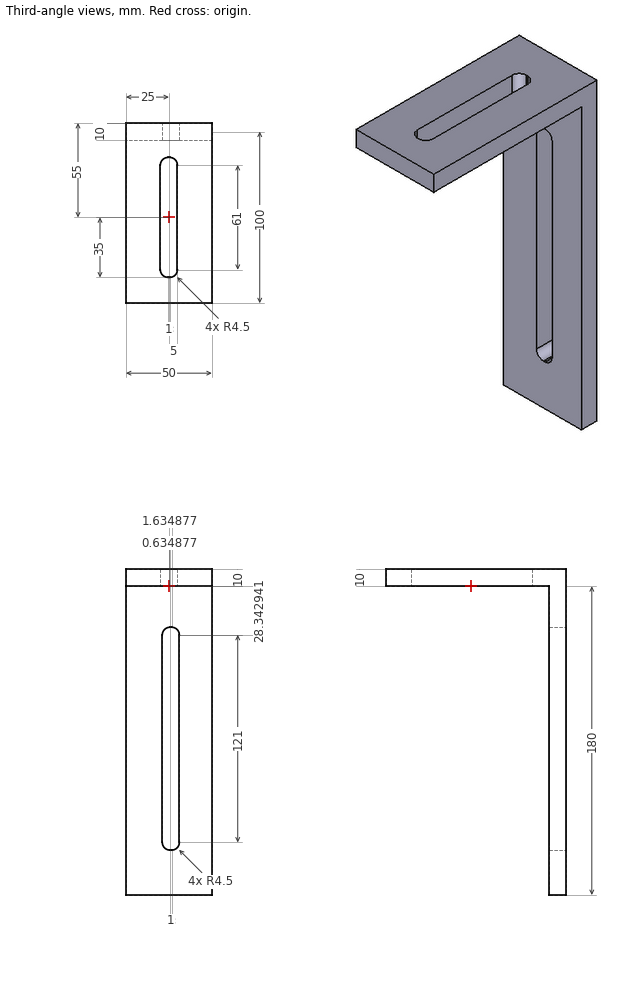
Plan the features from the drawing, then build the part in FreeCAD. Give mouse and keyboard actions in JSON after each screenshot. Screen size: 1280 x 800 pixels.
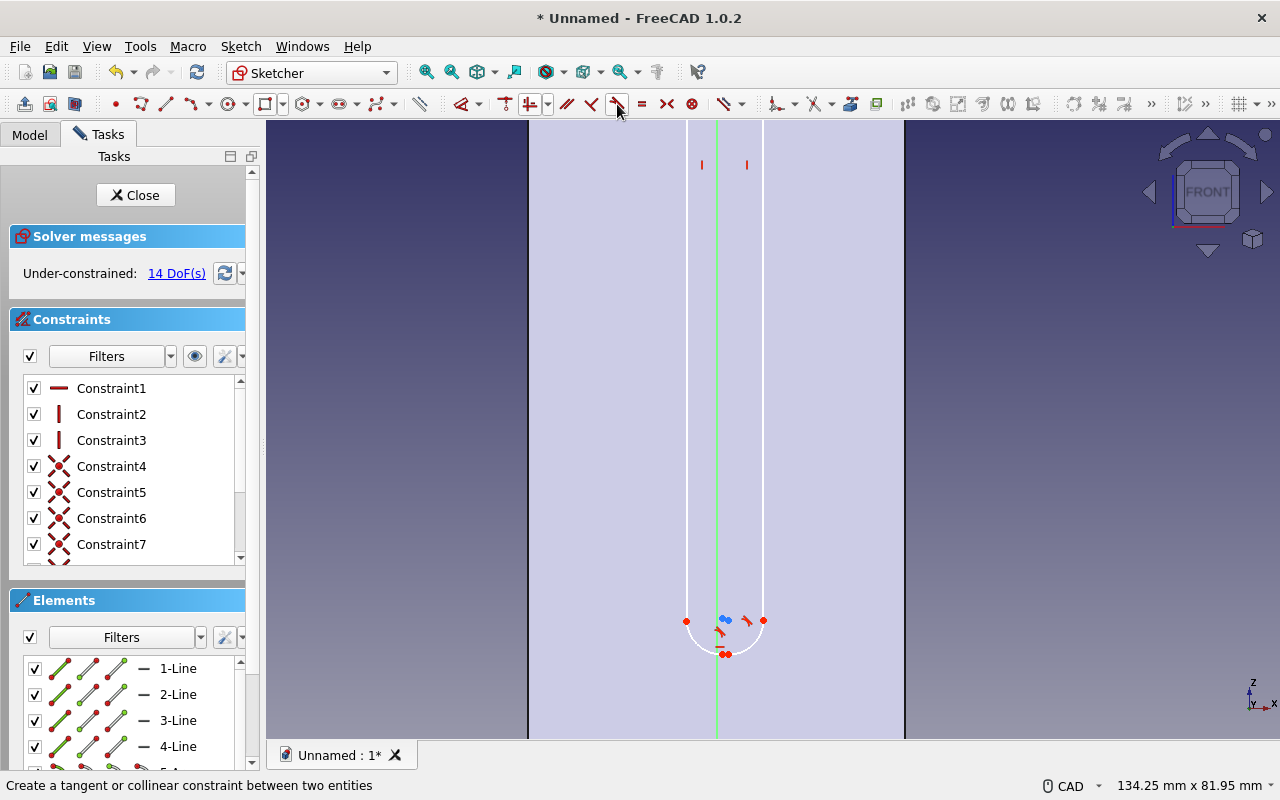
{"action": "left_click", "coordinate": [763, 347]}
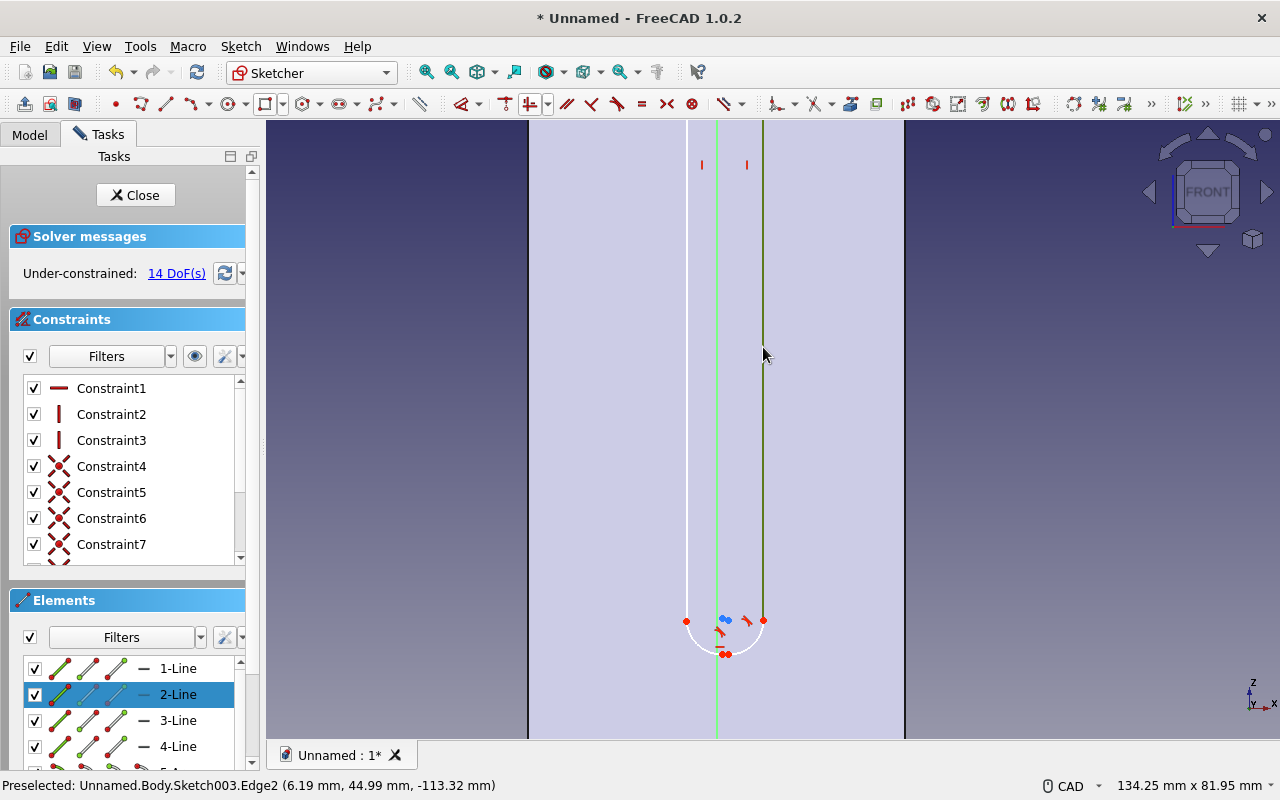
{"action": "scroll", "coordinate": [692, 637], "scroll_direction": "down", "scroll_amount": 5}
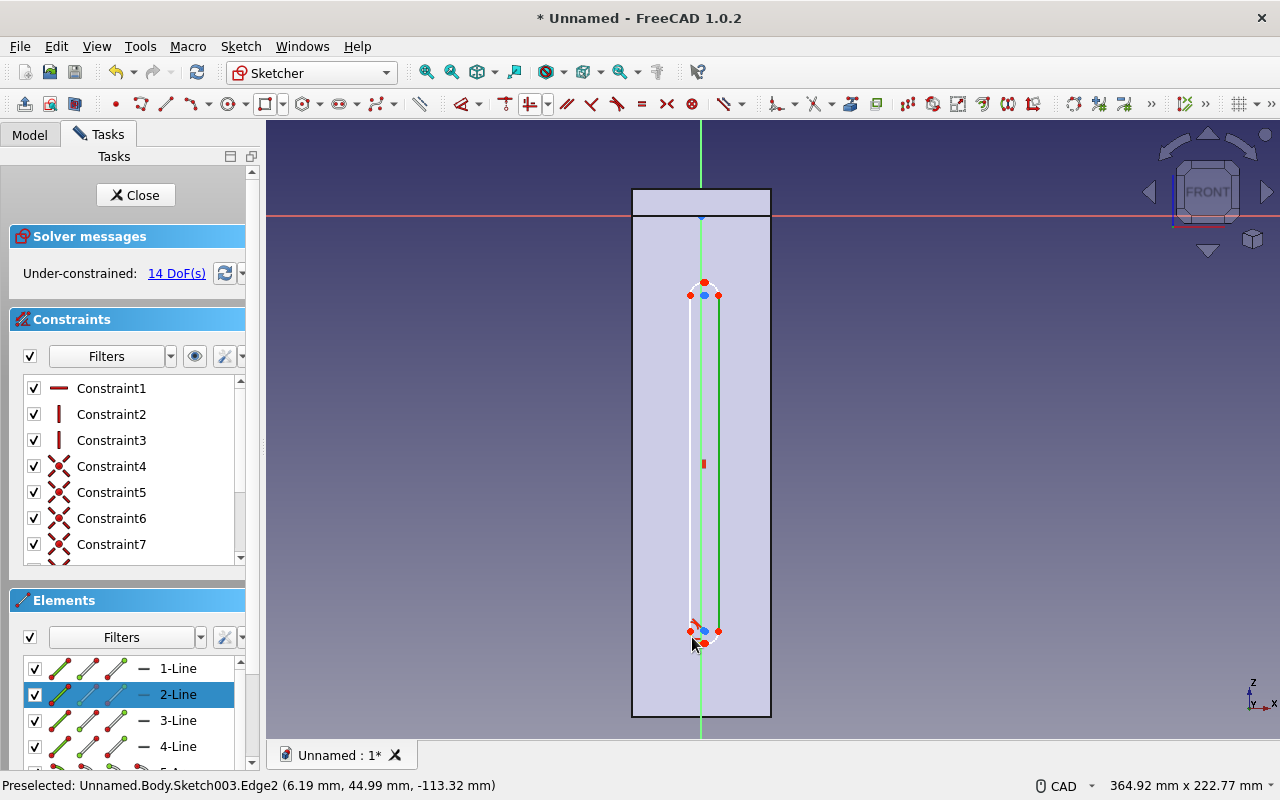
{"action": "scroll", "coordinate": [717, 290], "scroll_direction": "up", "scroll_amount": 5}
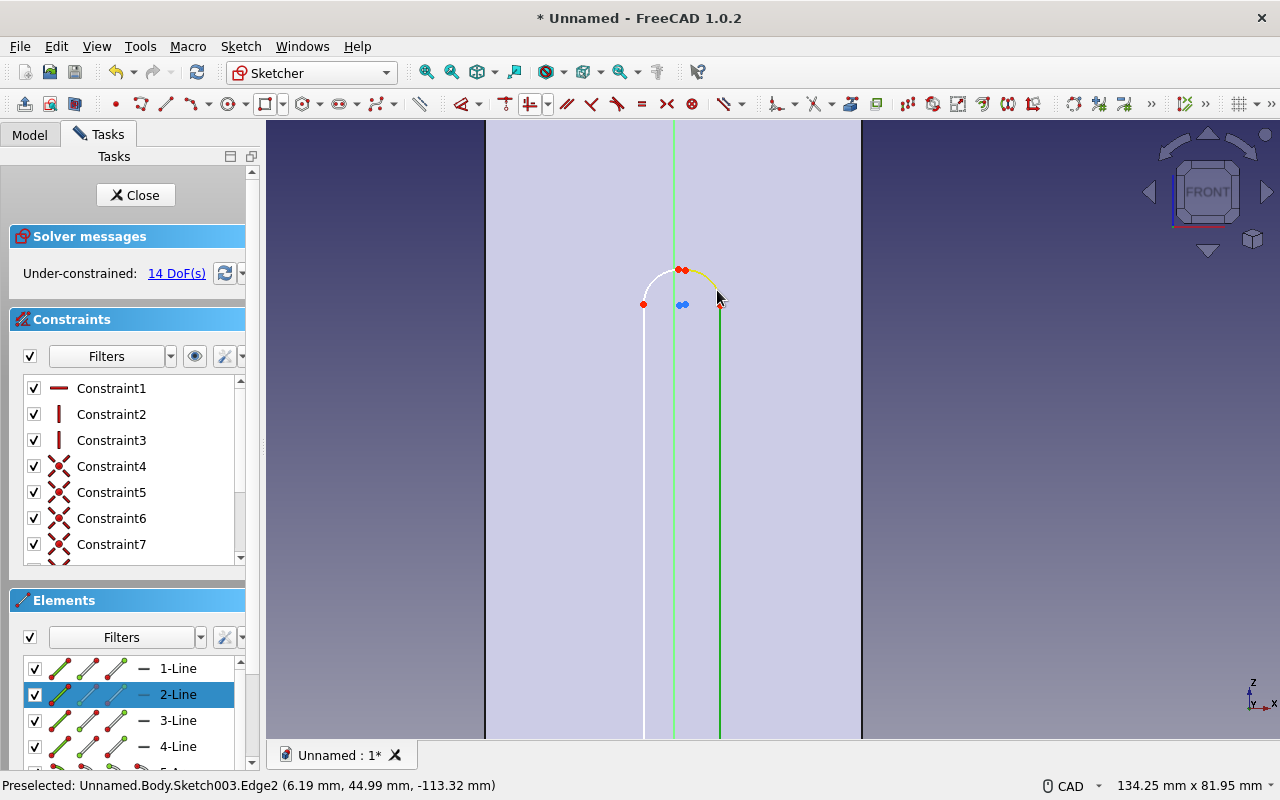
{"action": "left_click", "coordinate": [717, 290]}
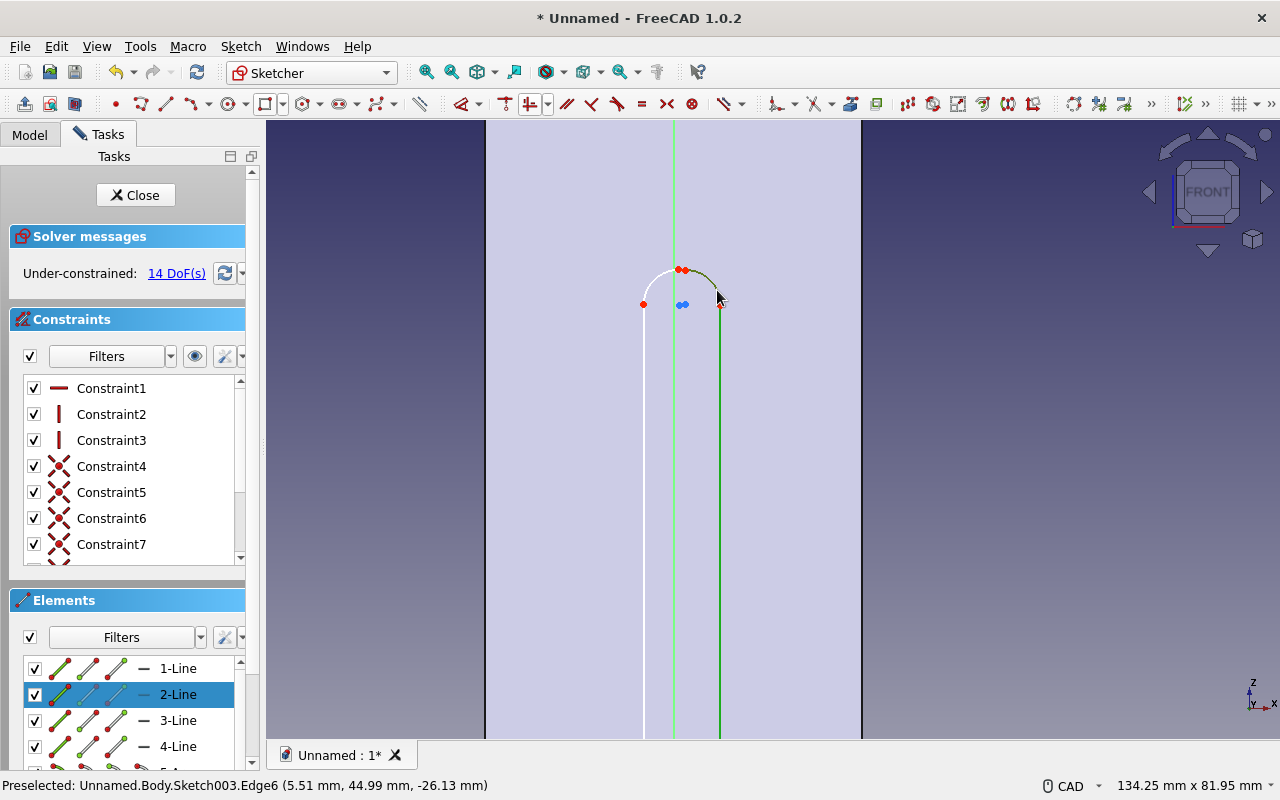
{"action": "left_click", "coordinate": [617, 104]}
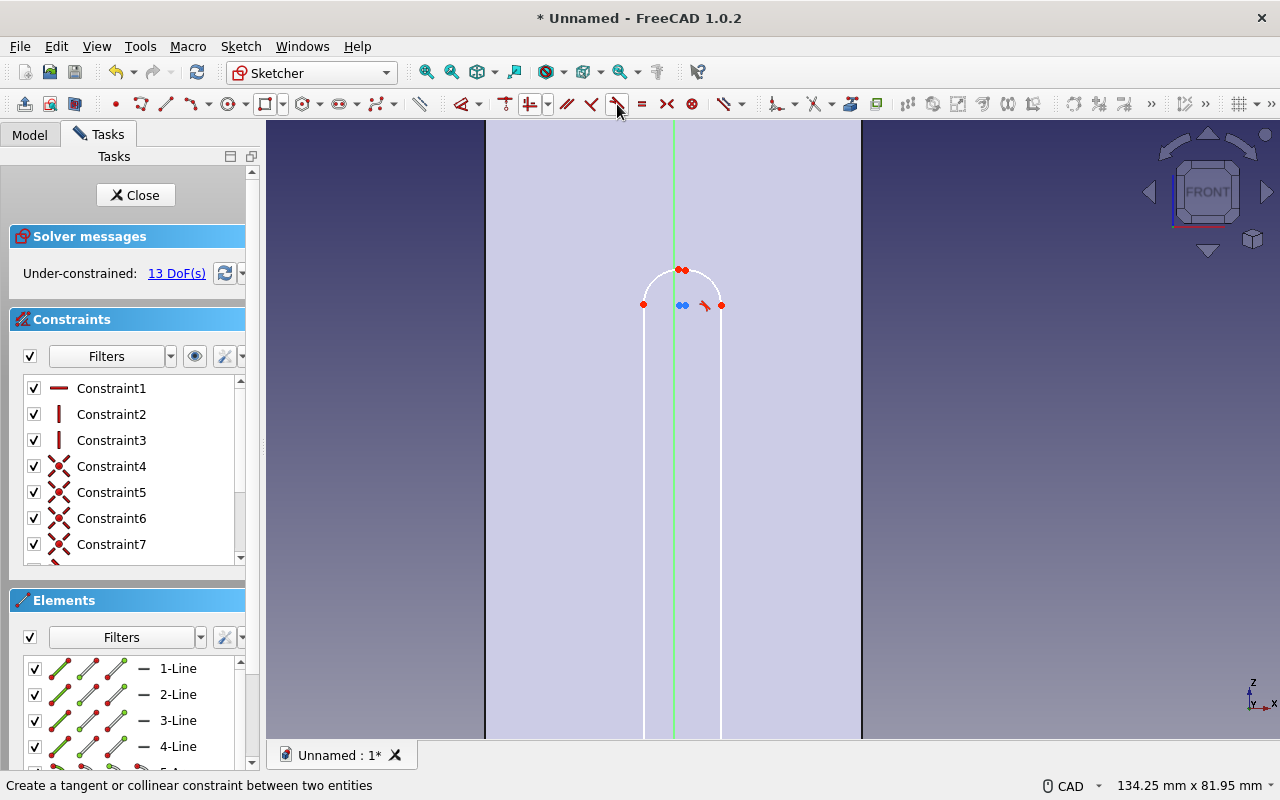
{"action": "scroll", "coordinate": [682, 270], "scroll_direction": "up", "scroll_amount": 7}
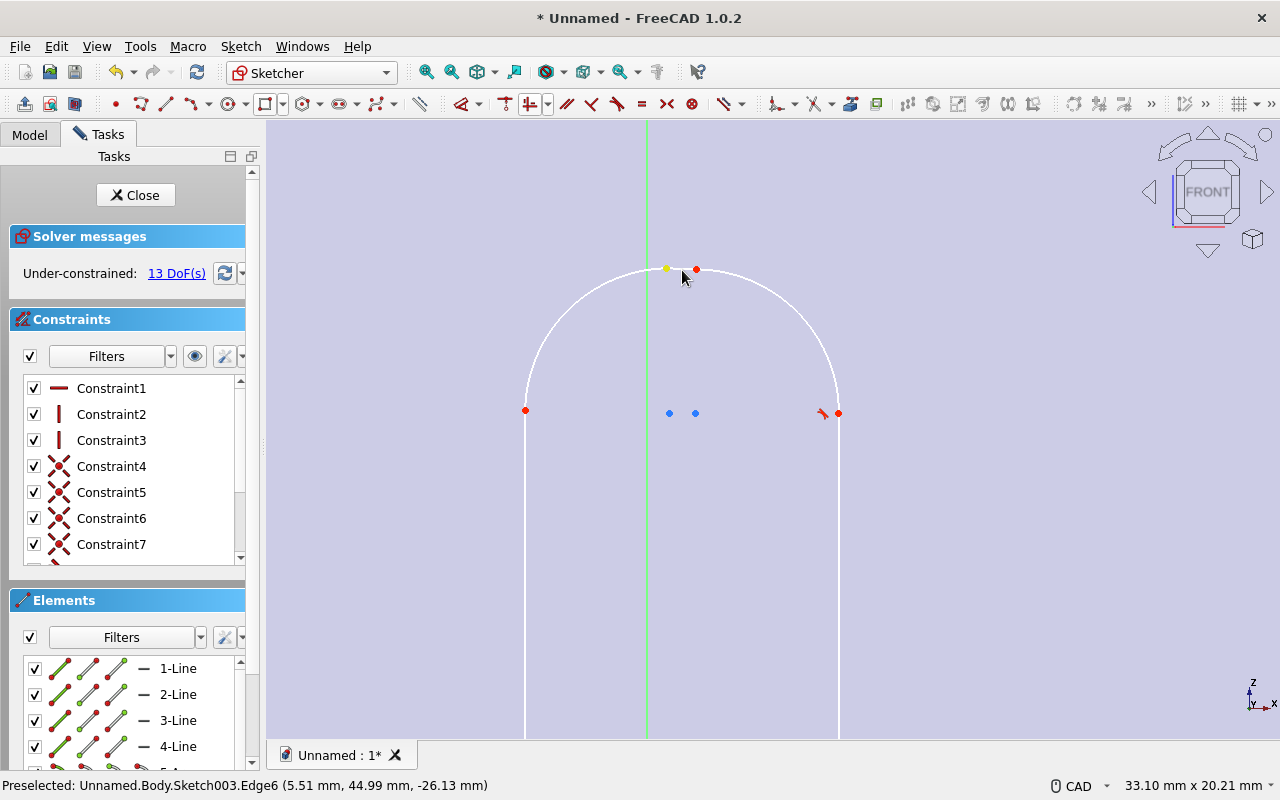
{"action": "left_click", "coordinate": [682, 269]}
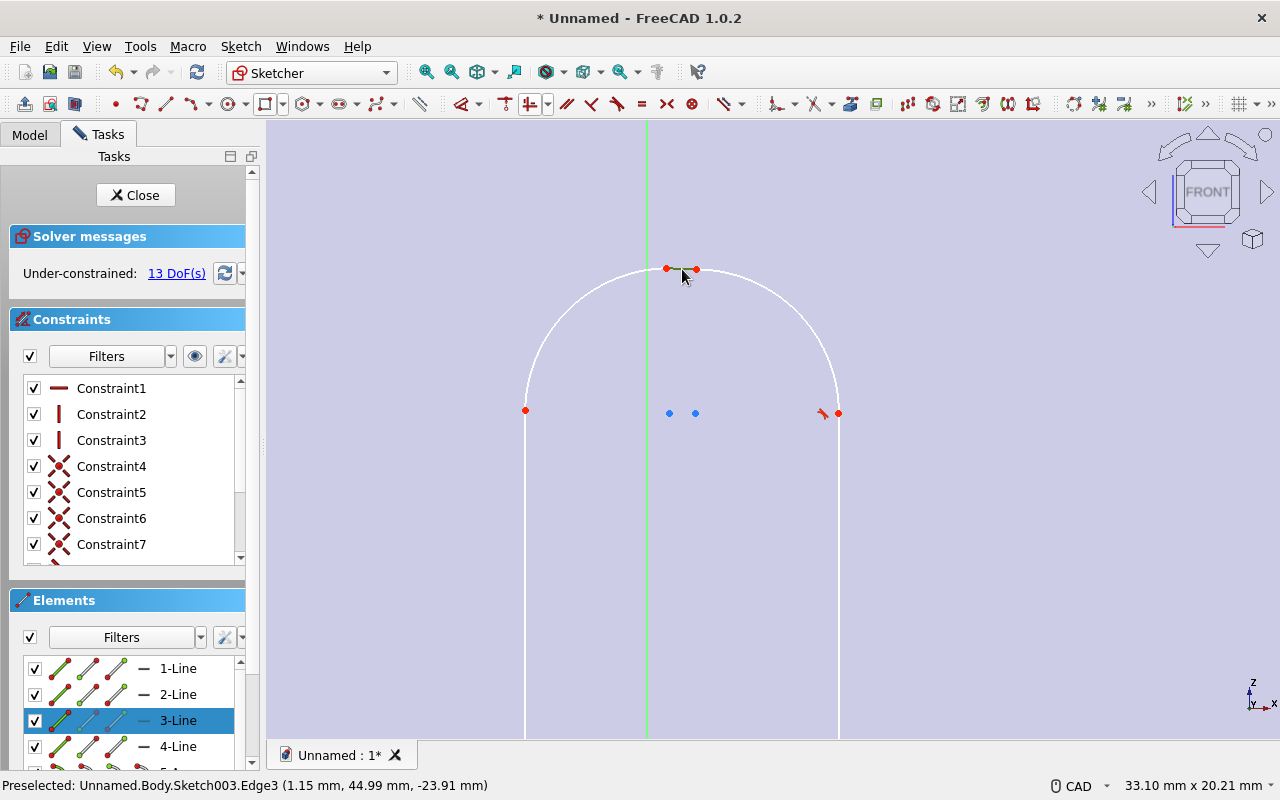
{"action": "scroll", "coordinate": [707, 284], "scroll_direction": "down", "scroll_amount": 12}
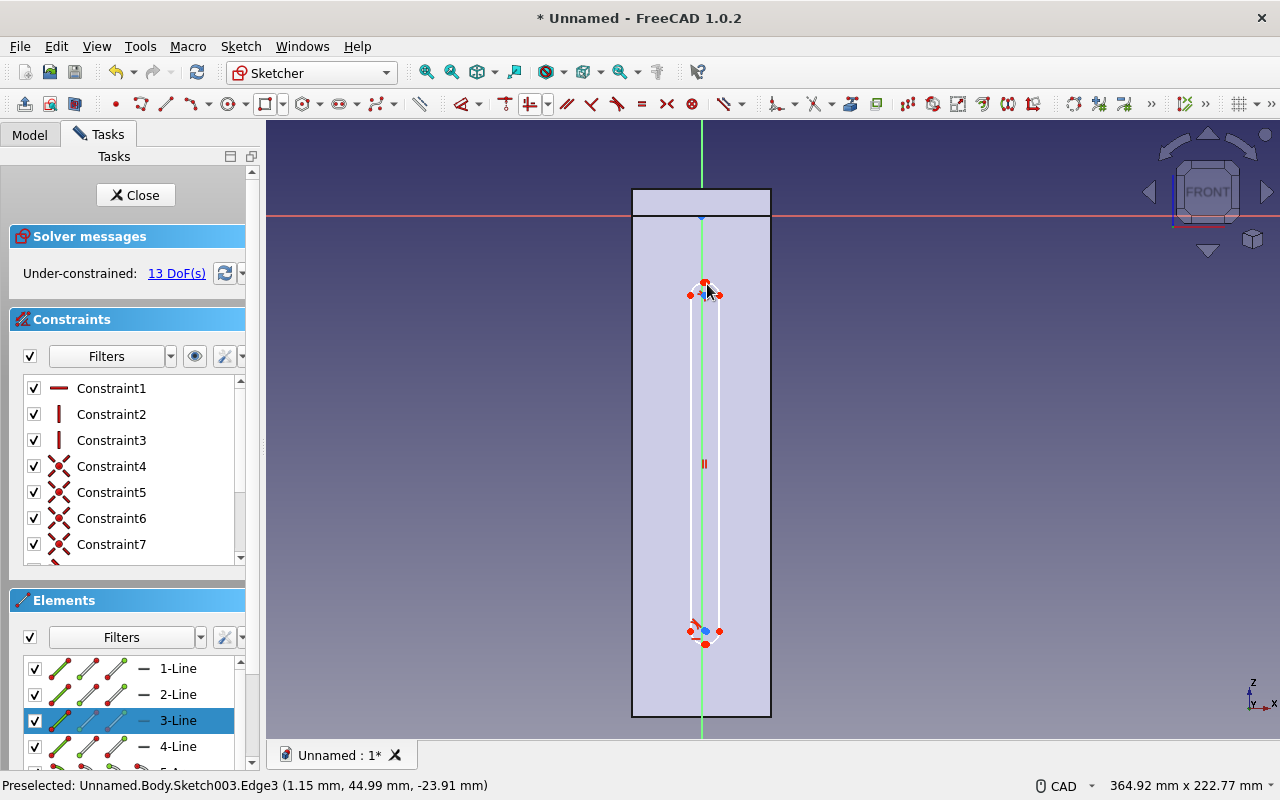
{"action": "scroll", "coordinate": [718, 290], "scroll_direction": "up", "scroll_amount": 5}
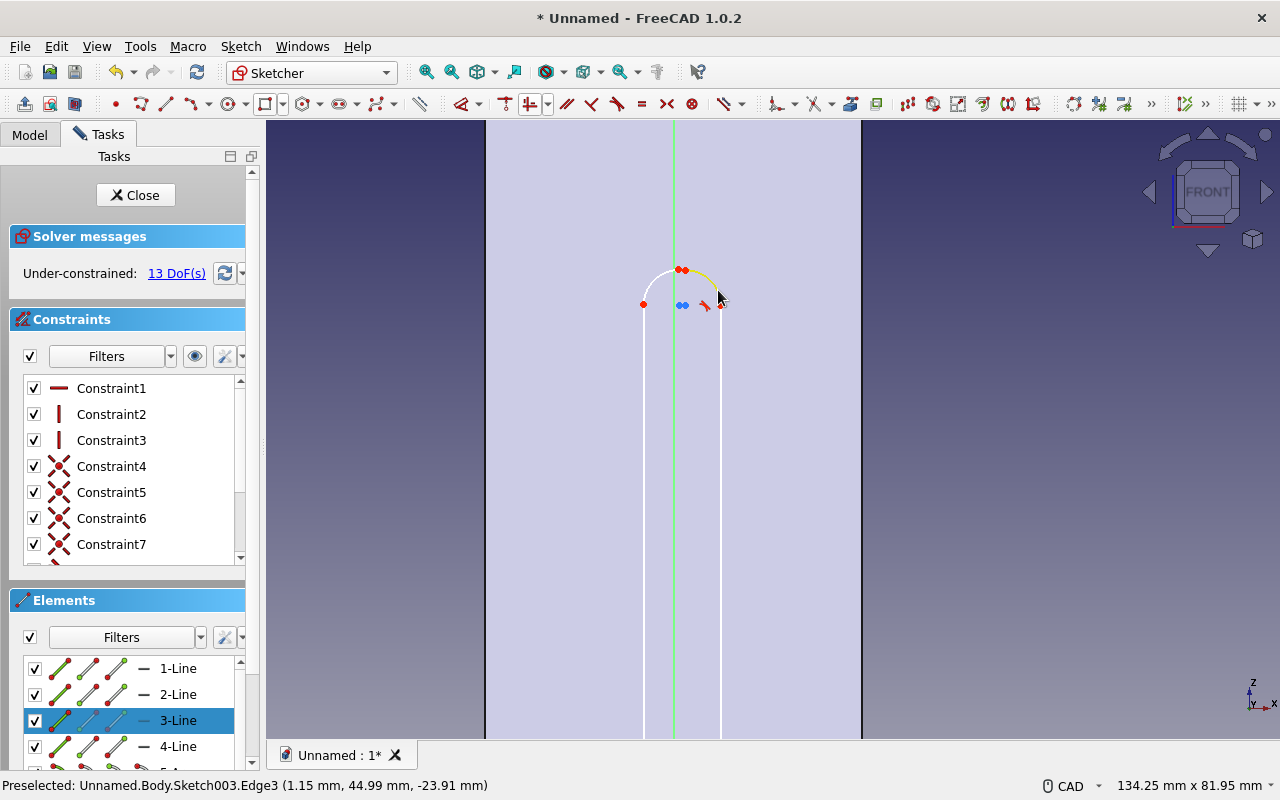
{"action": "left_click", "coordinate": [717, 290]}